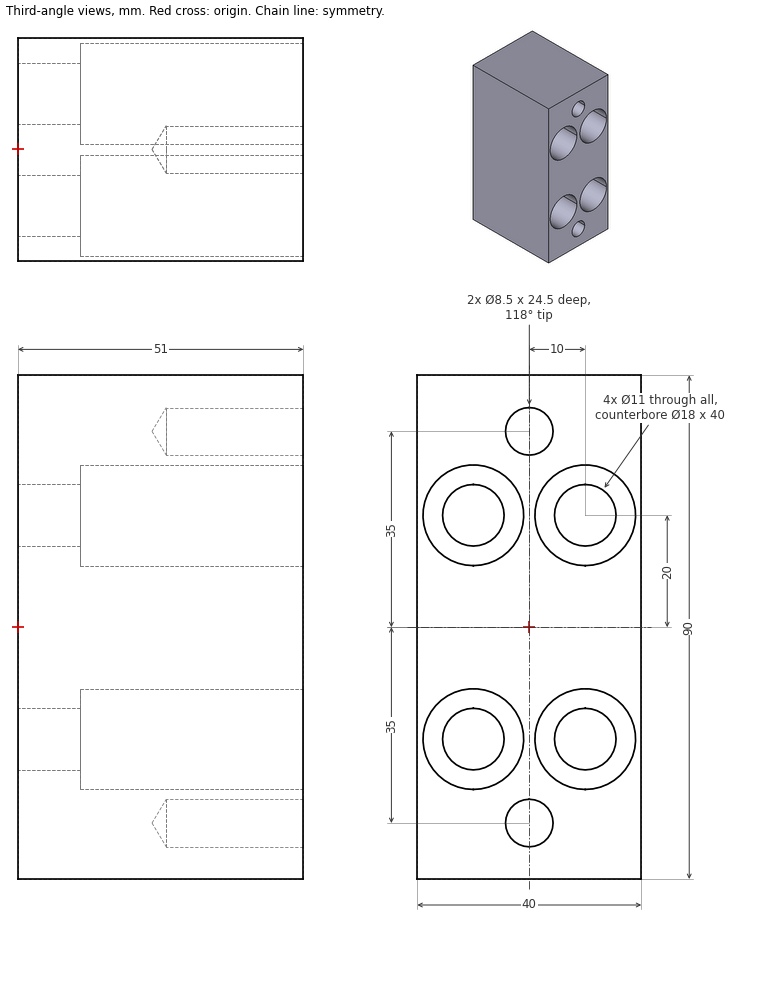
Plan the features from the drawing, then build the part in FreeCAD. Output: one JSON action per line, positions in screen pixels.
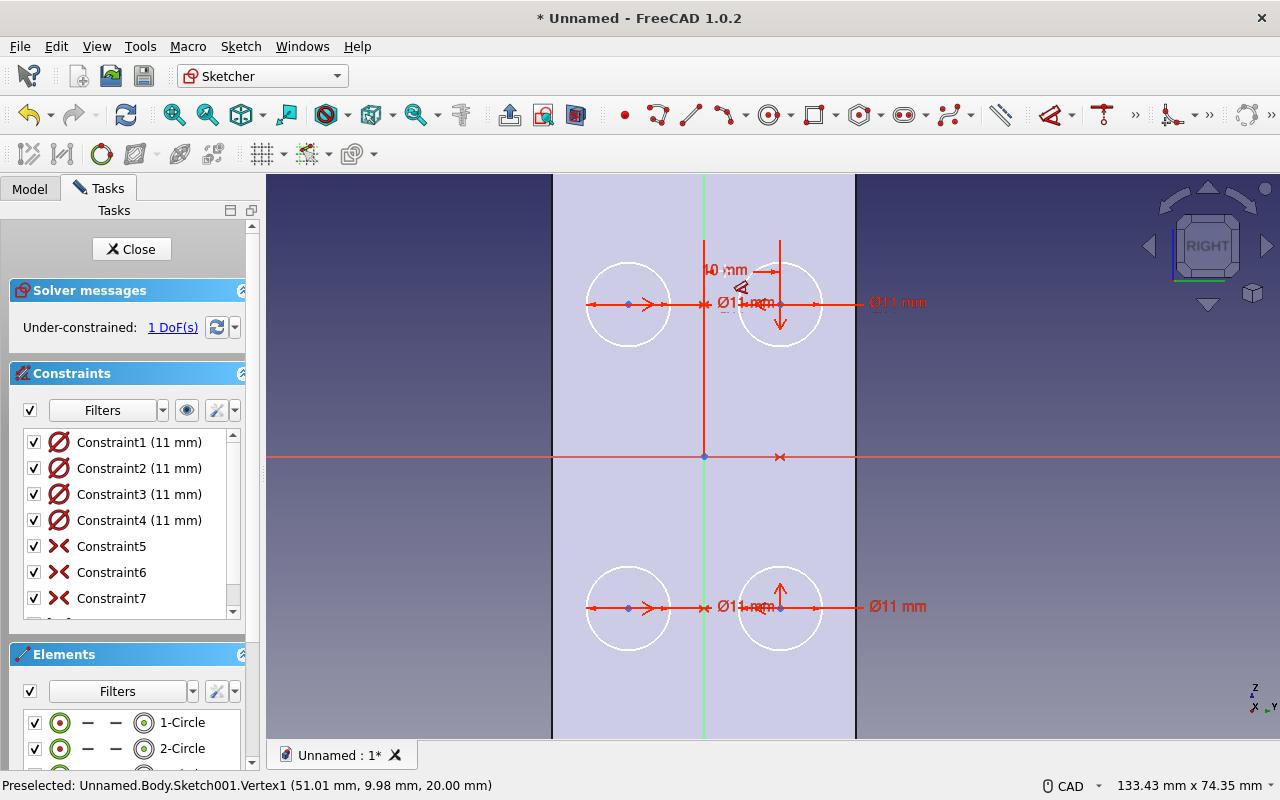
{"action": "left_click", "coordinate": [780, 305]}
{"action": "left_click", "coordinate": [814, 381]}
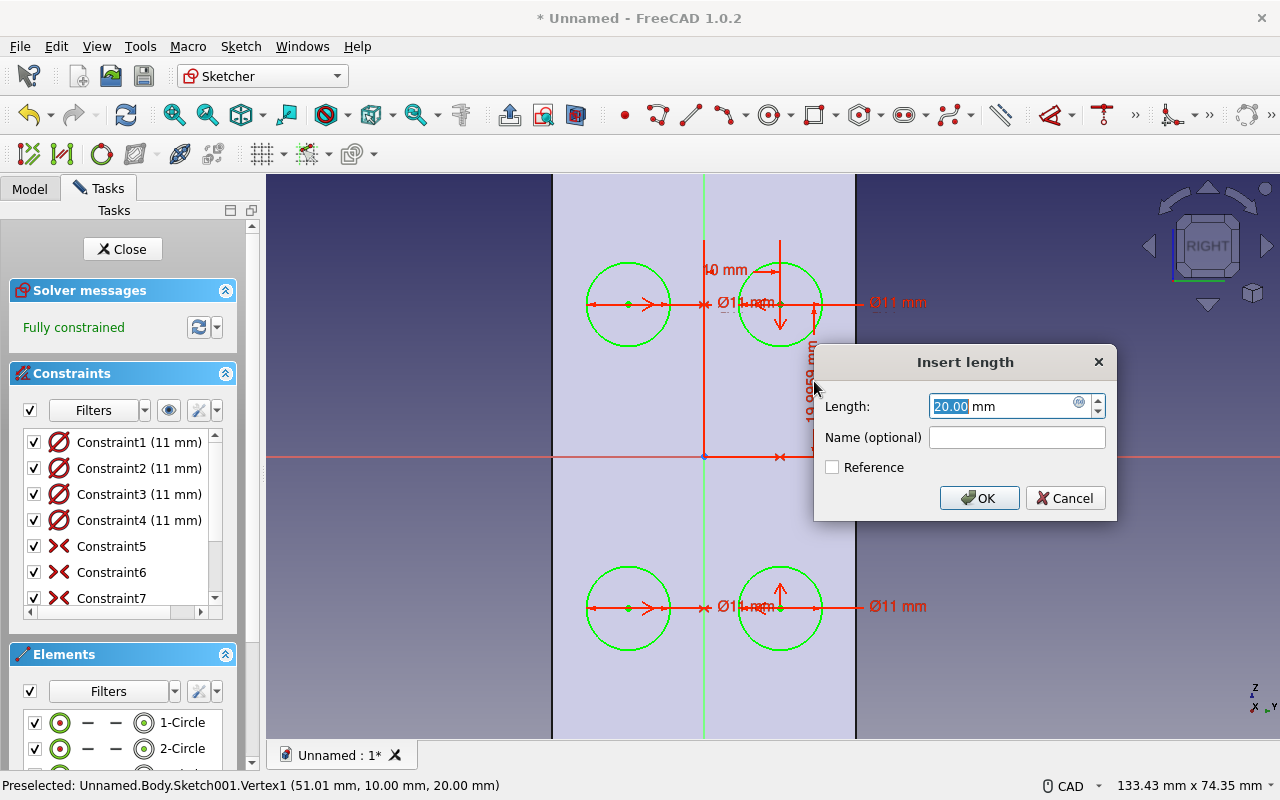
{"action": "type", "text": "20"}
{"action": "key", "text": "Return"}
{"action": "key", "text": "Escape"}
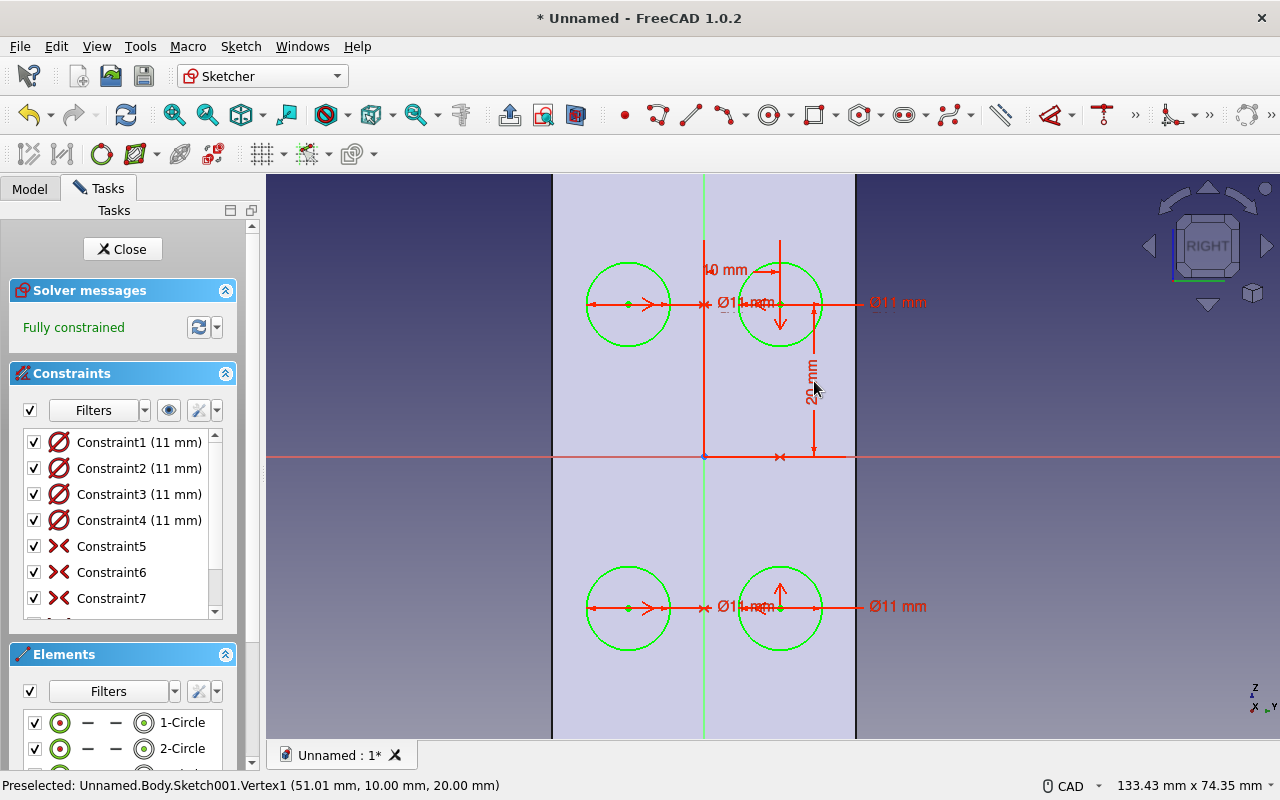
{"action": "left_click", "coordinate": [123, 249]}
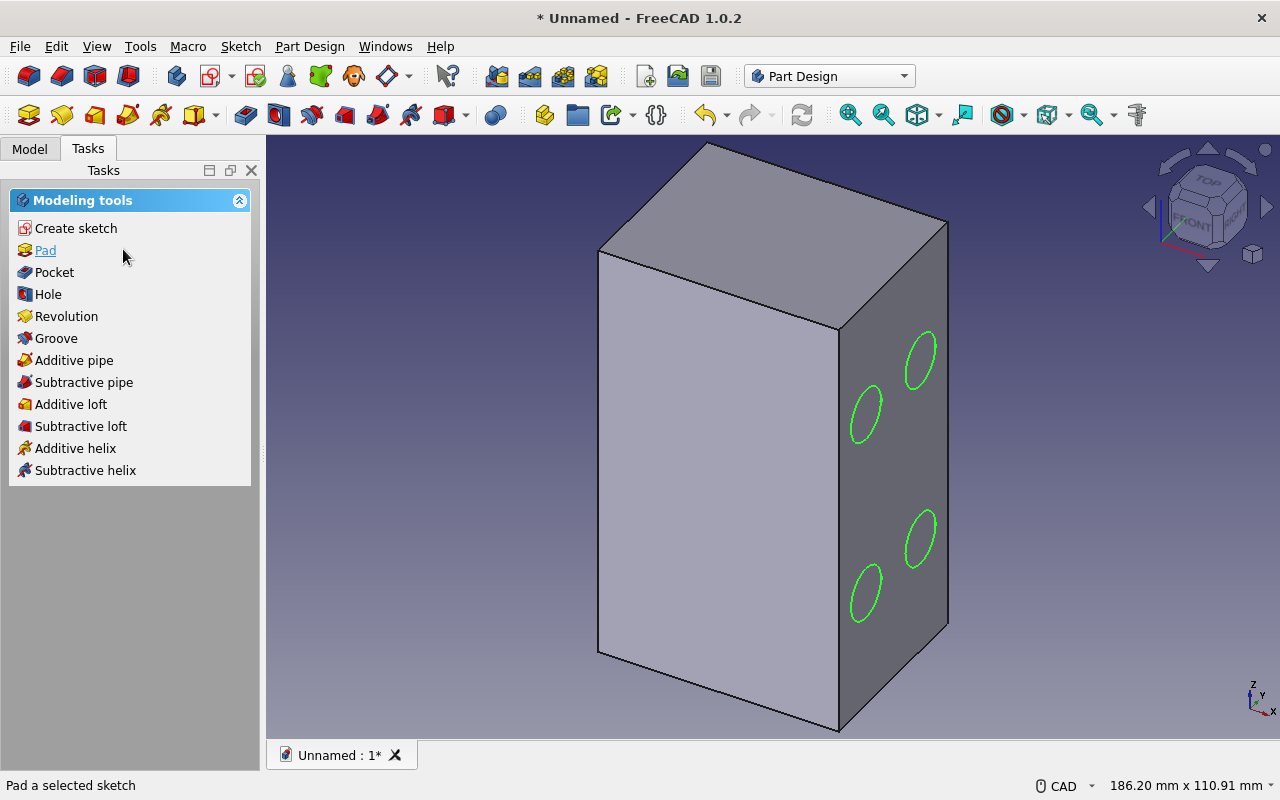
{"action": "left_click", "coordinate": [279, 116]}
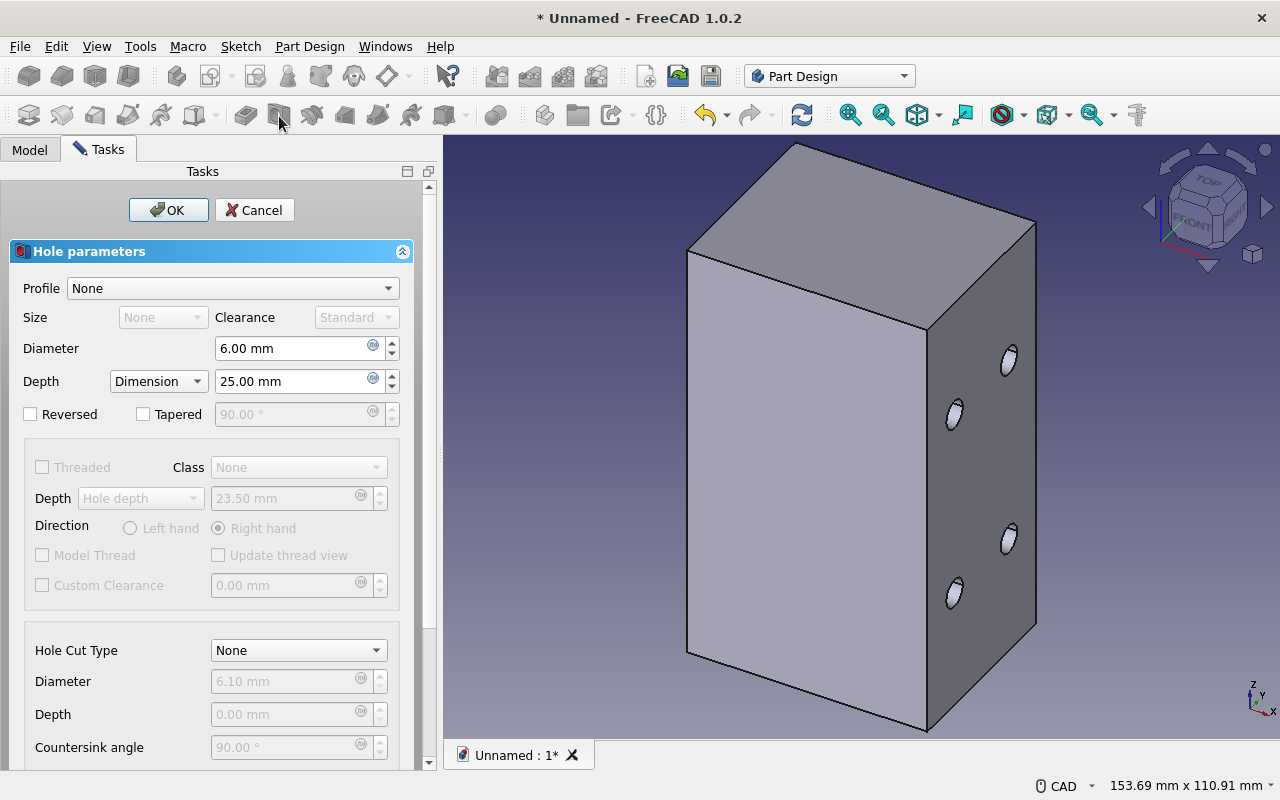
{"action": "triple_click", "coordinate": [300, 348]}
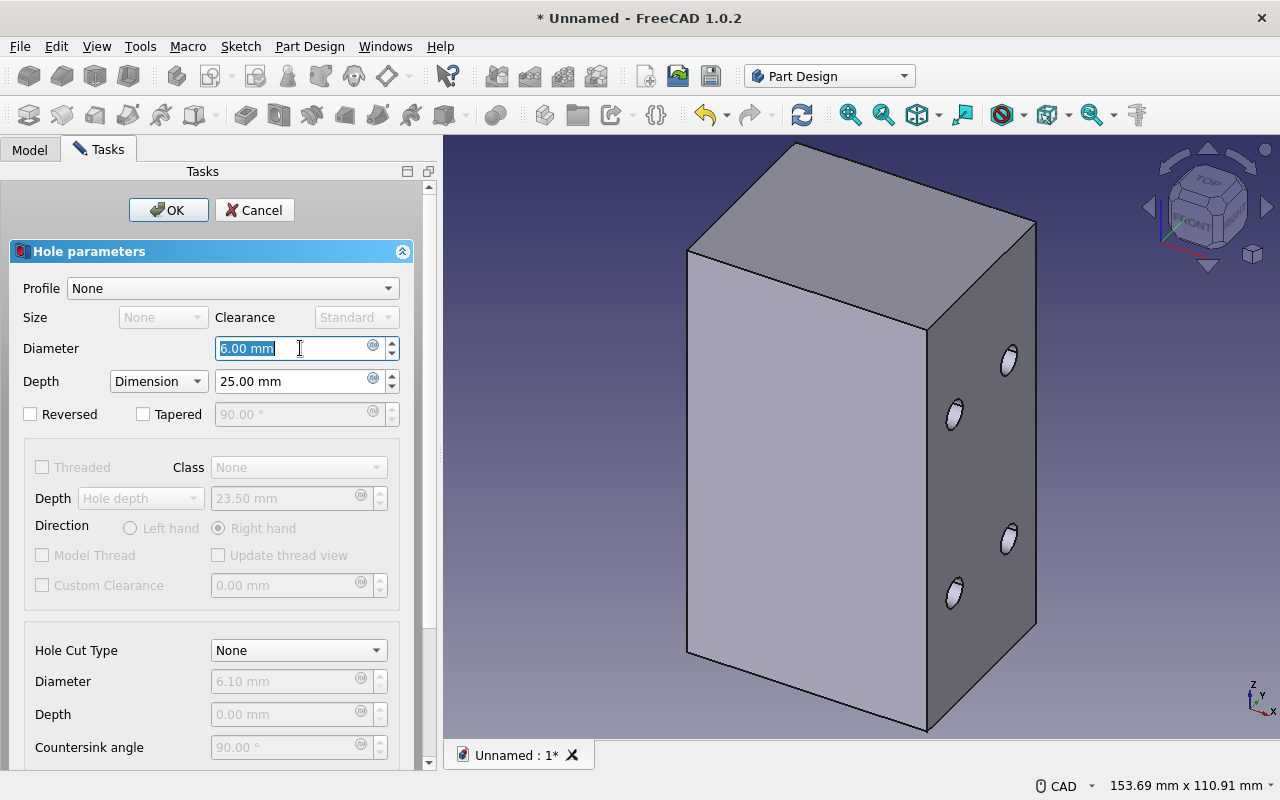
{"action": "type", "text": "11"}
{"action": "key", "text": "Tab"}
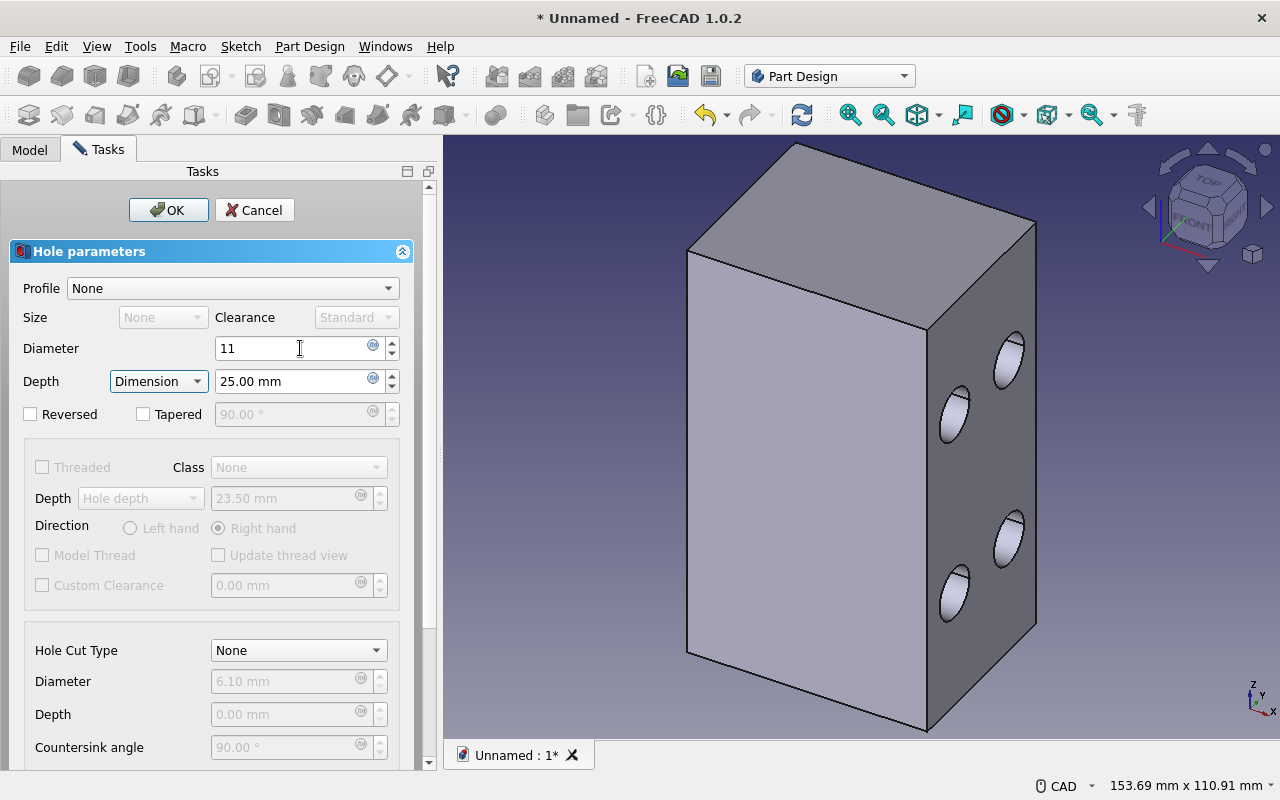
{"action": "left_click", "coordinate": [160, 382]}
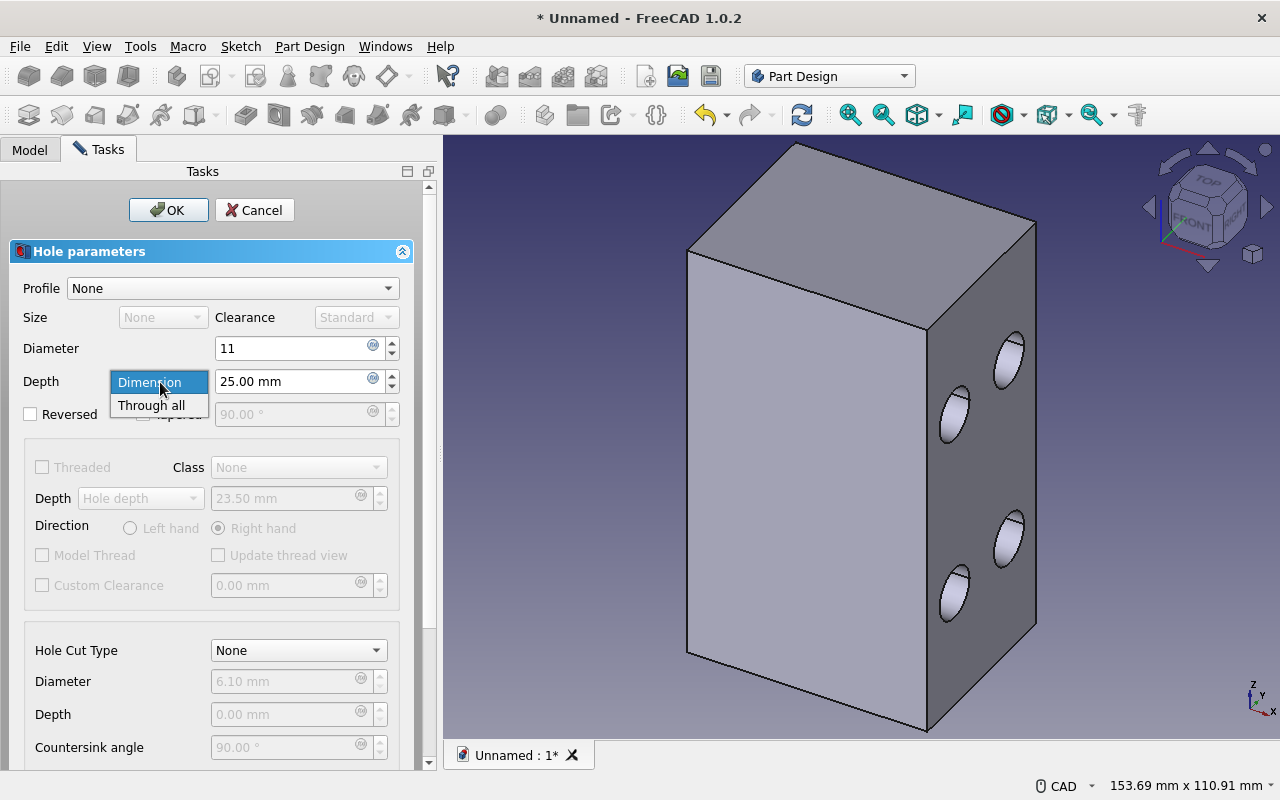
{"action": "left_click", "coordinate": [158, 406]}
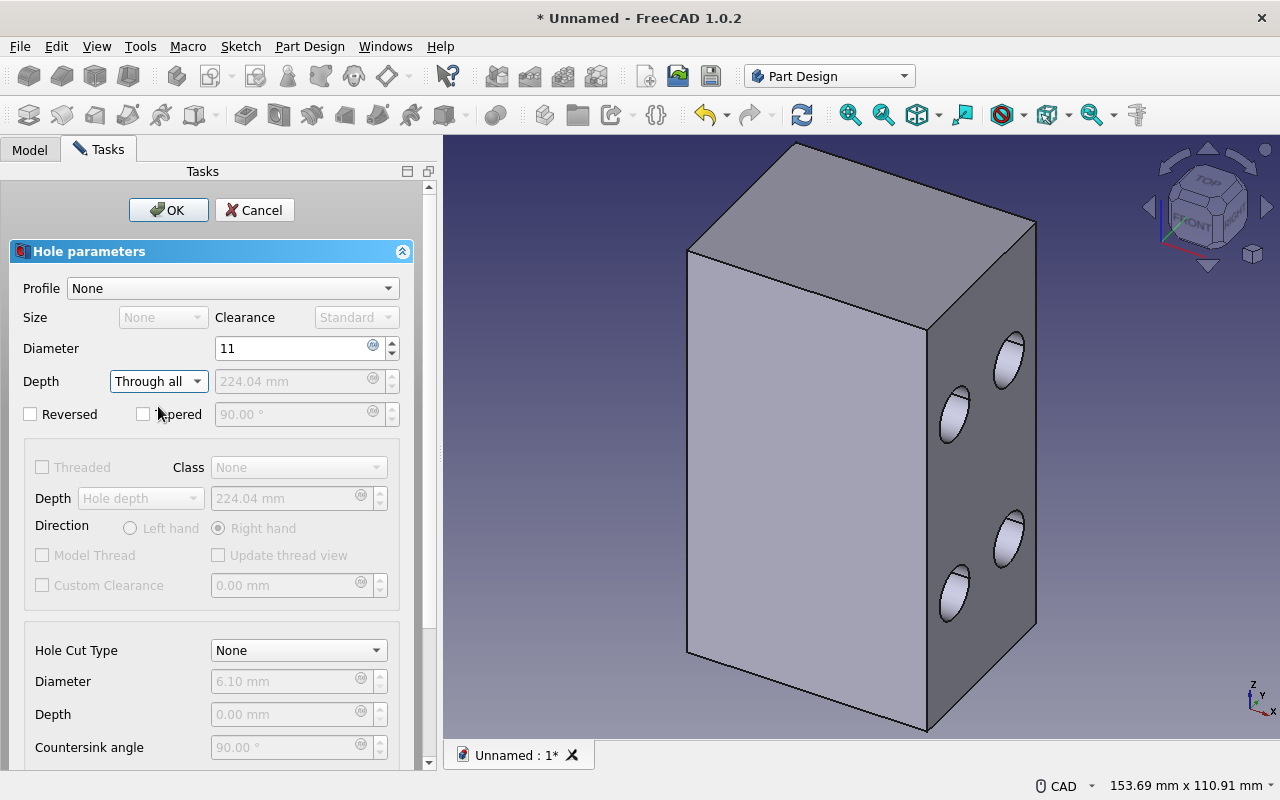
{"action": "left_click", "coordinate": [300, 650]}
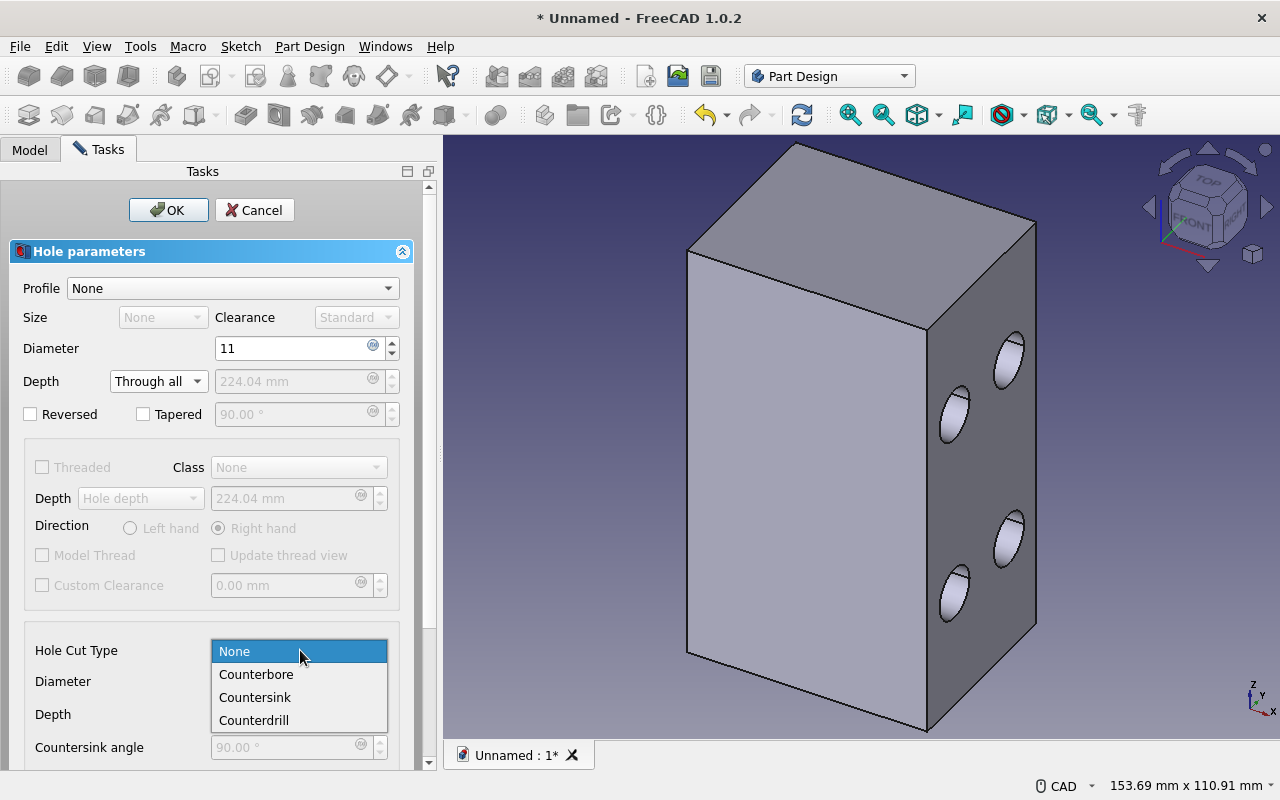
{"action": "left_click", "coordinate": [298, 674]}